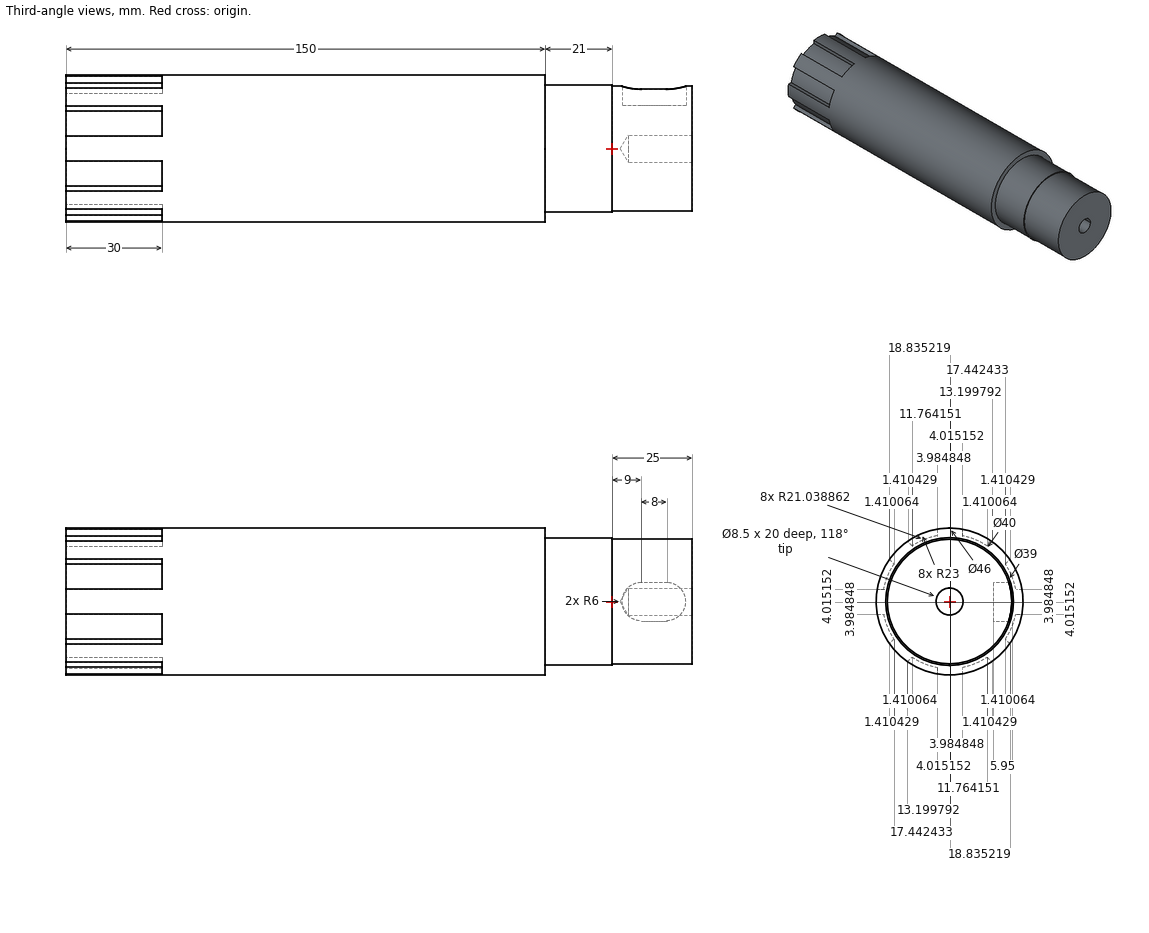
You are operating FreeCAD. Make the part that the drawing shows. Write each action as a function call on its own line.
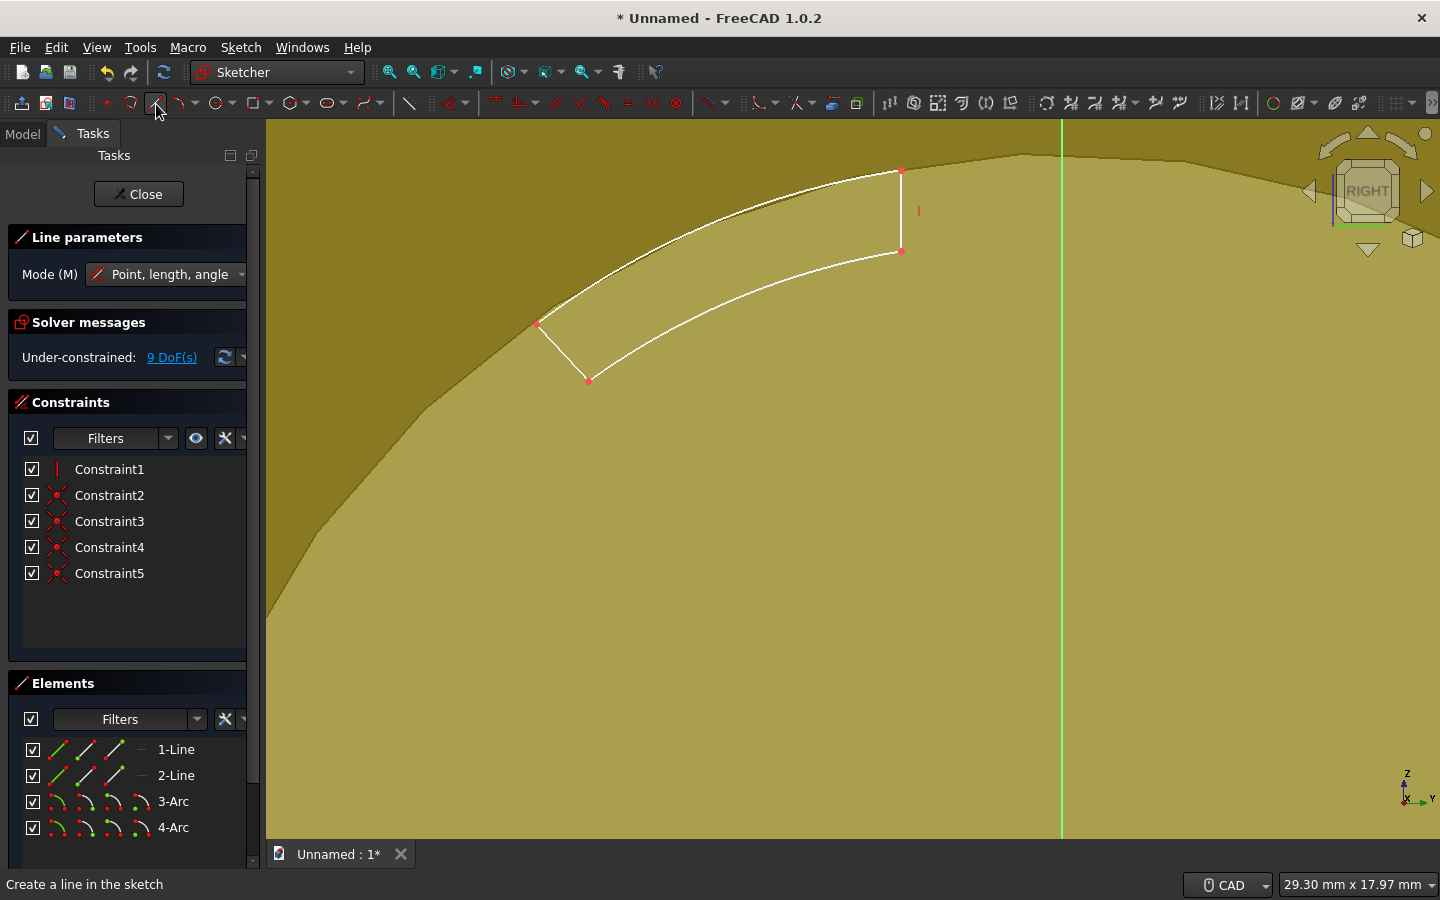
scroll(694, 284, down, 7)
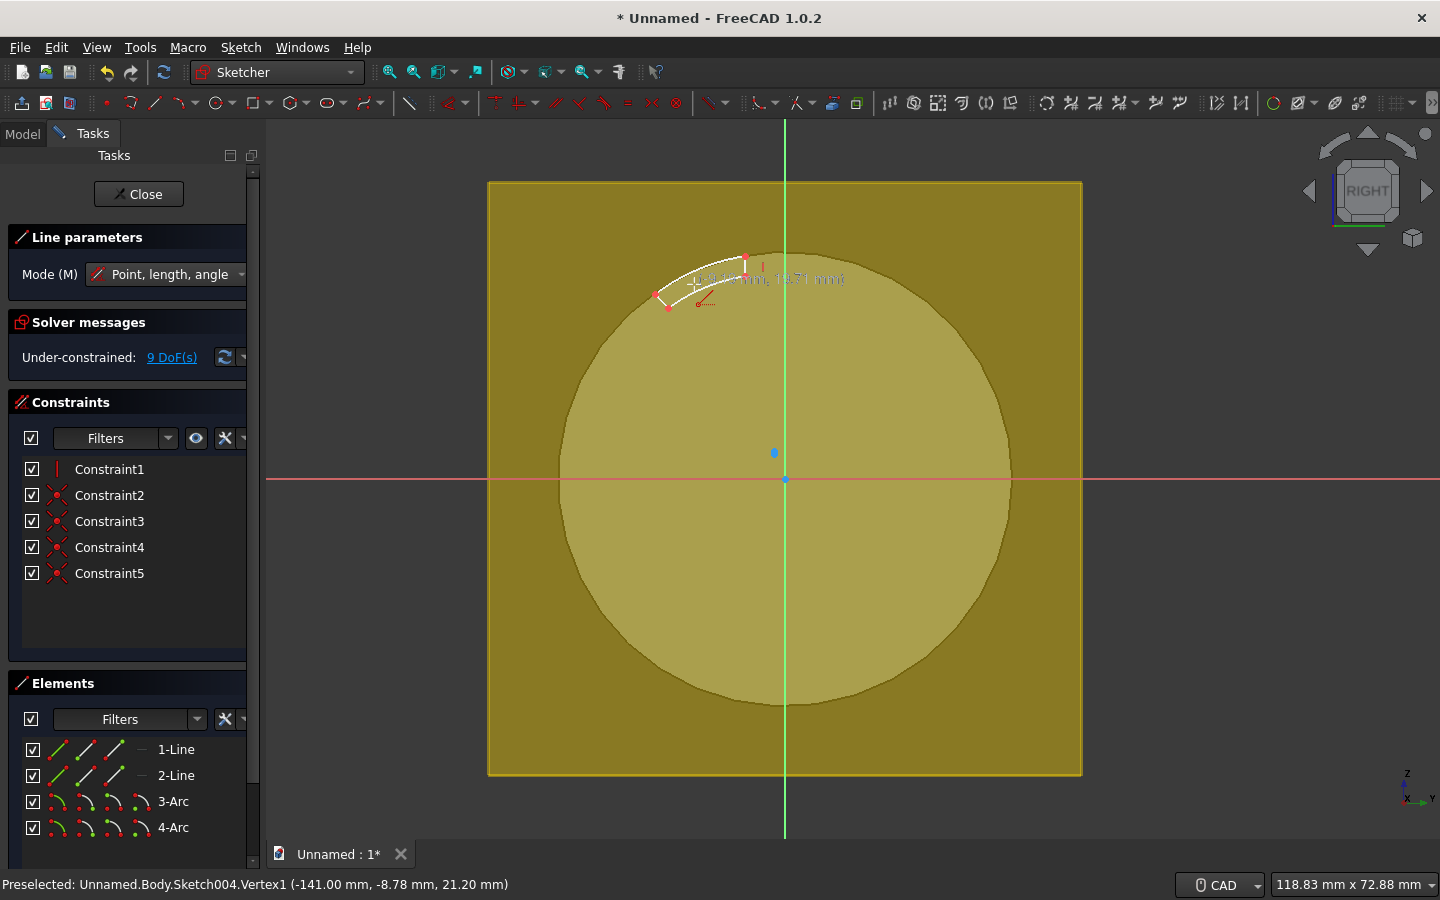
click(915, 293)
click(902, 307)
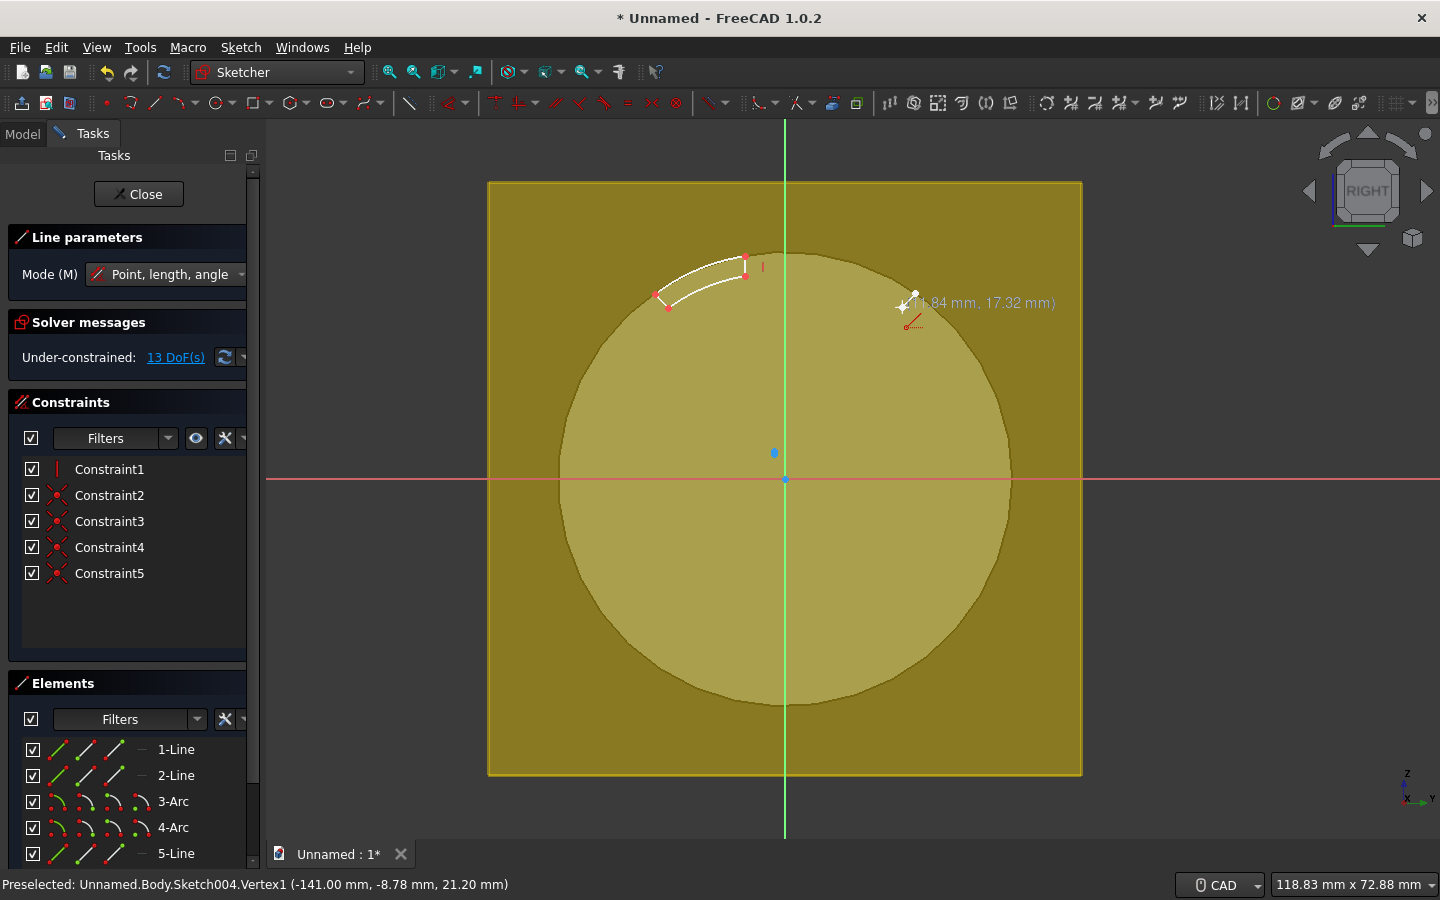
click(825, 275)
click(825, 255)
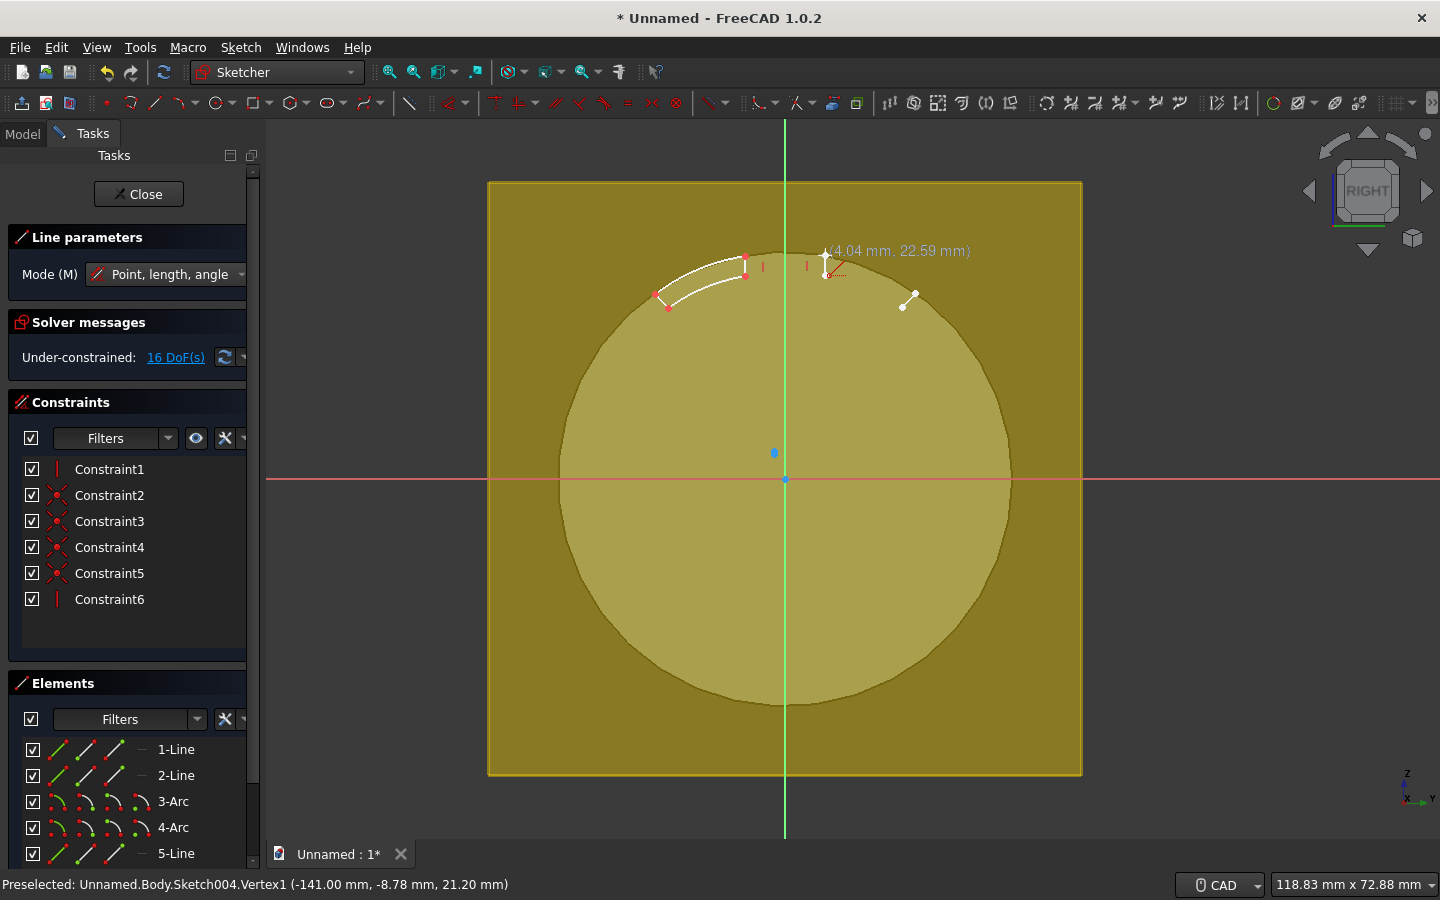
click(180, 104)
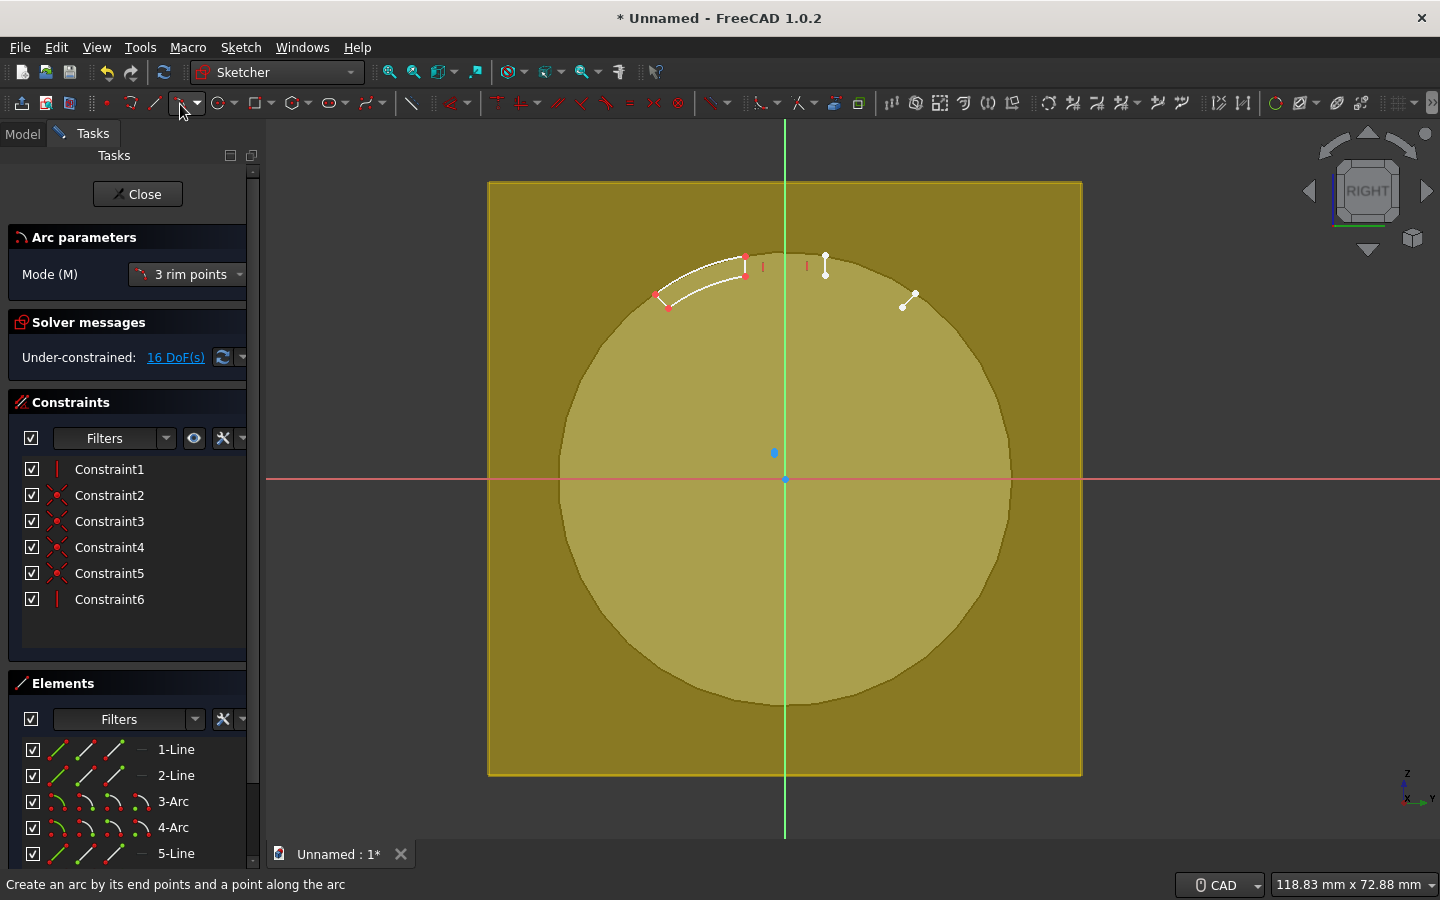
scroll(902, 307, up, 3)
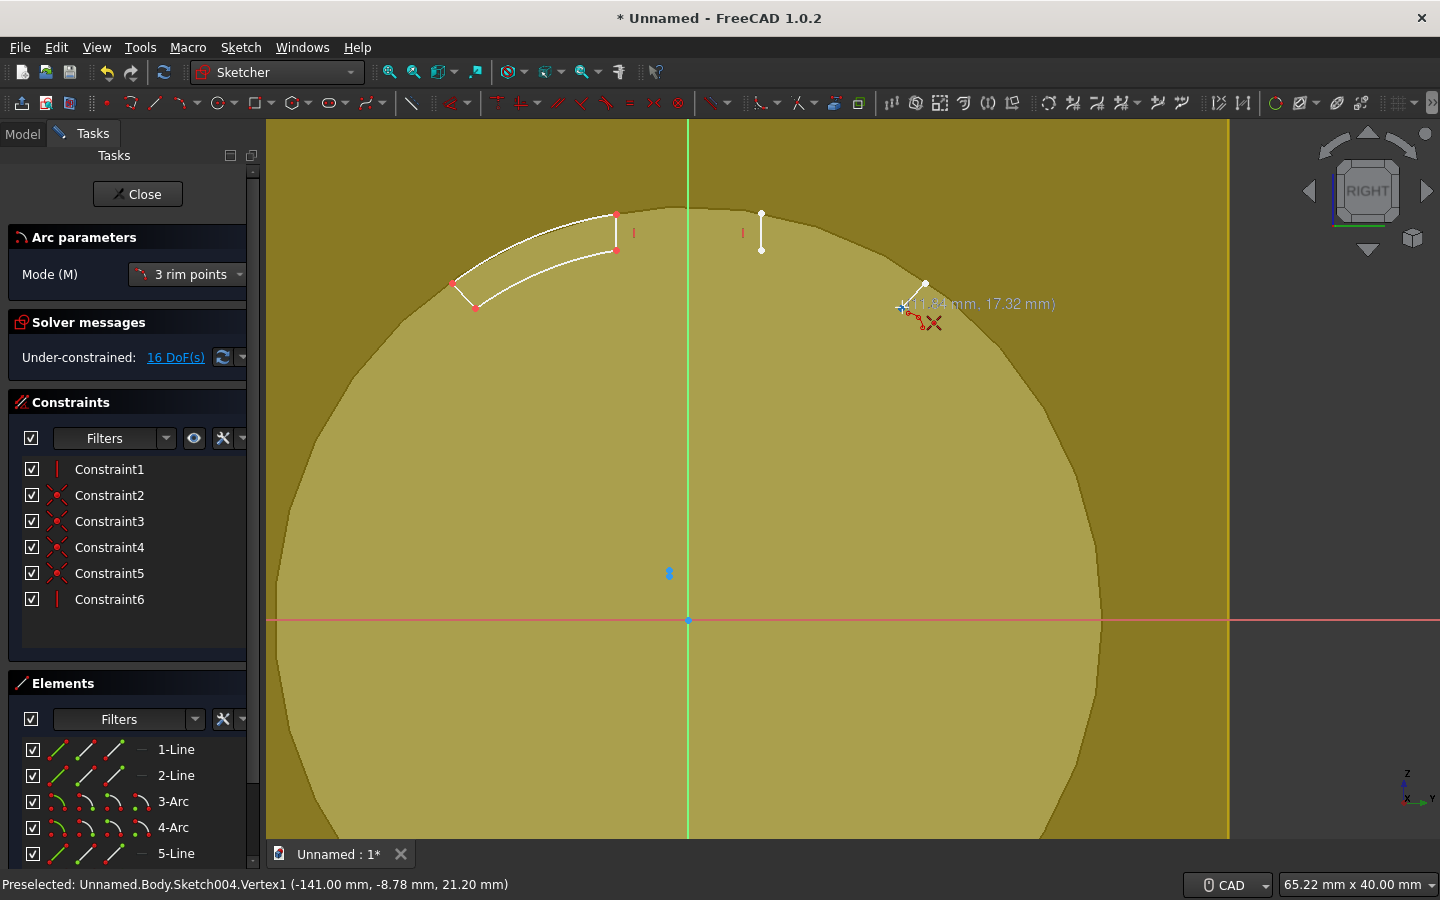
click(902, 309)
click(761, 250)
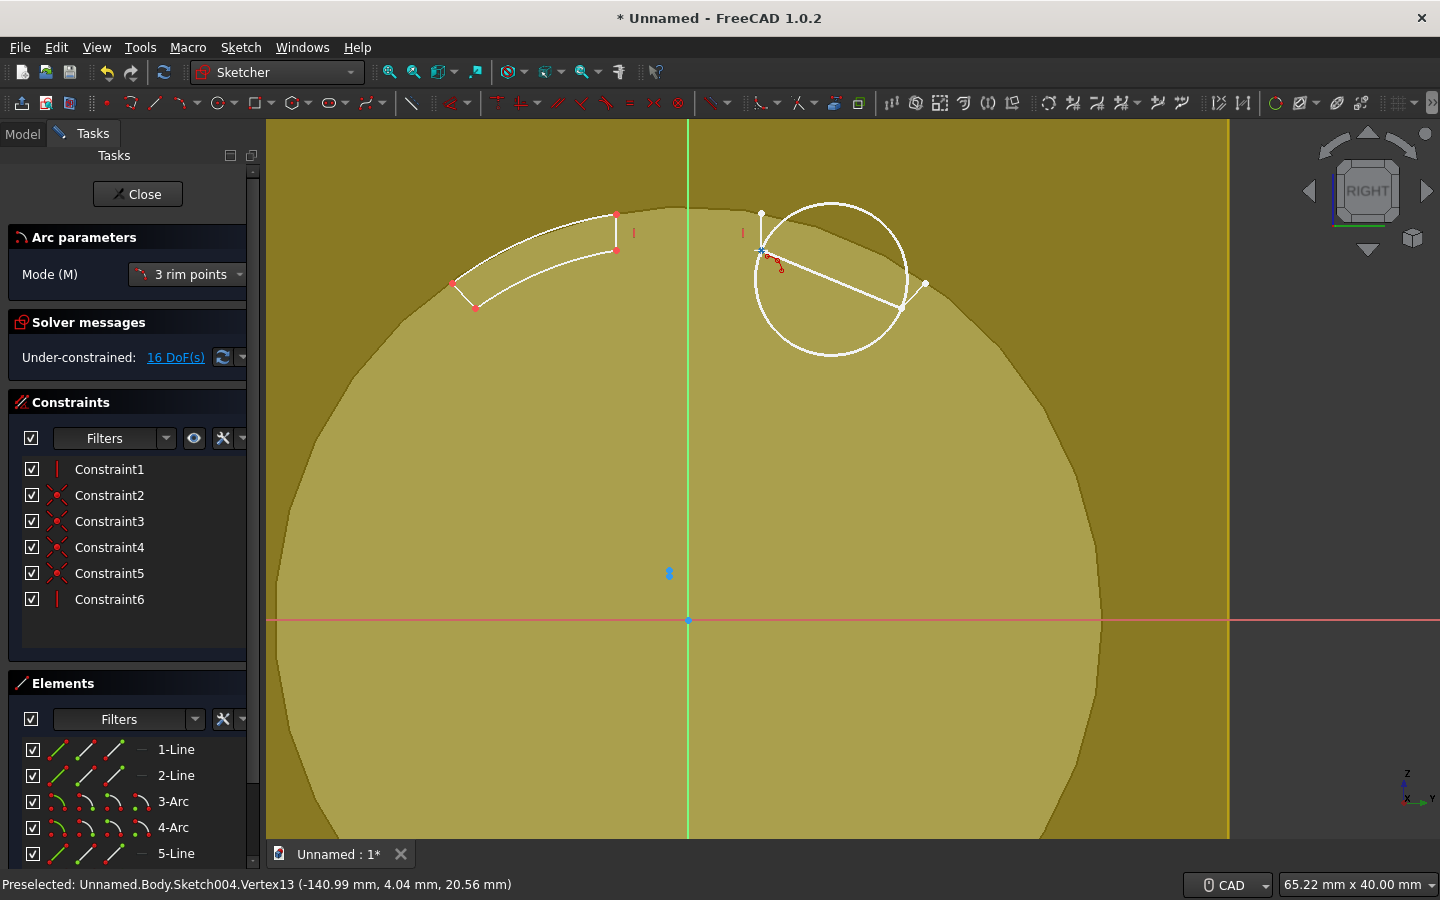
scroll(834, 271, up, 4)